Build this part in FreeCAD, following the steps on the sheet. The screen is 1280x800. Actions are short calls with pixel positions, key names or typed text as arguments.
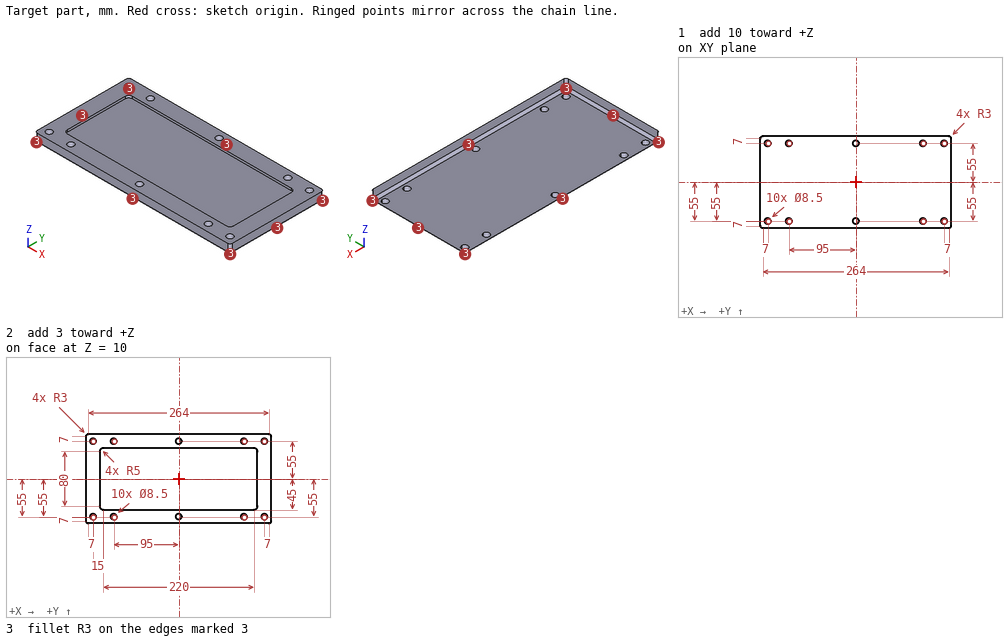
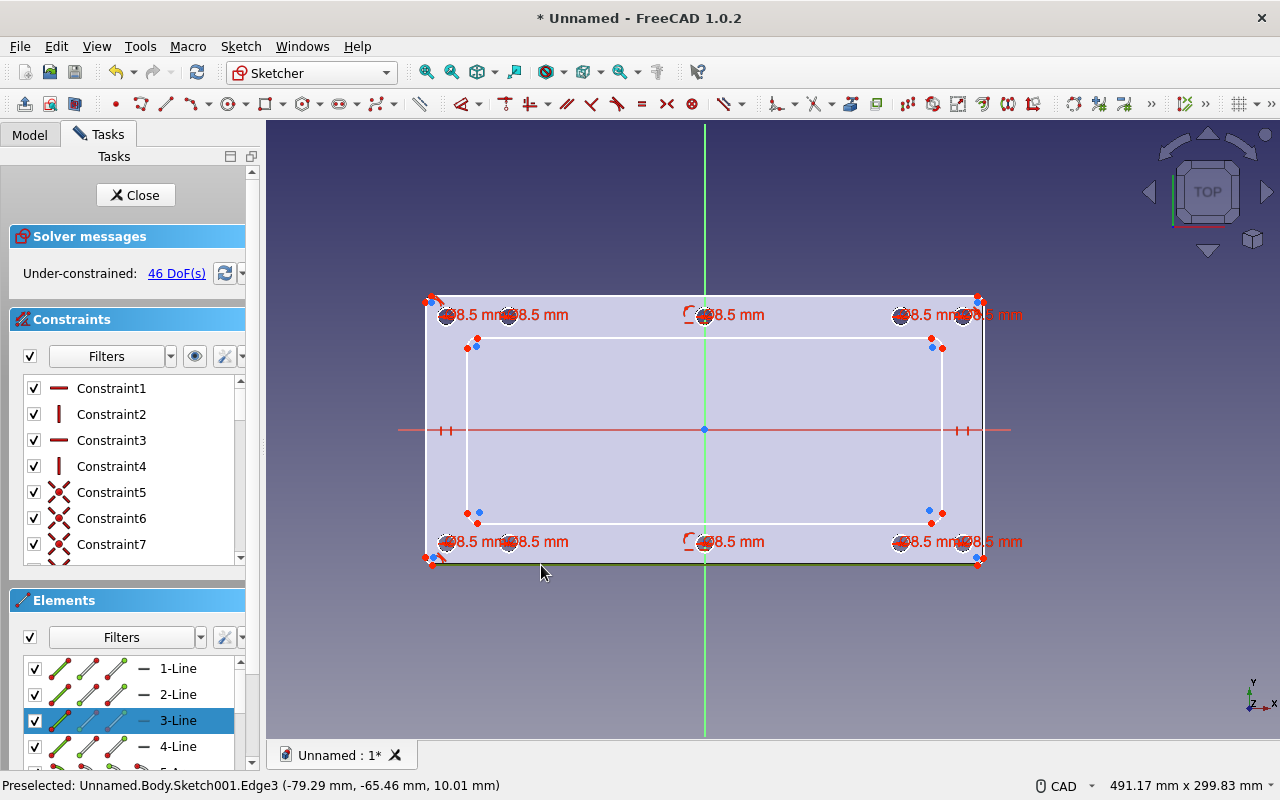
scroll(428, 563, up, 5)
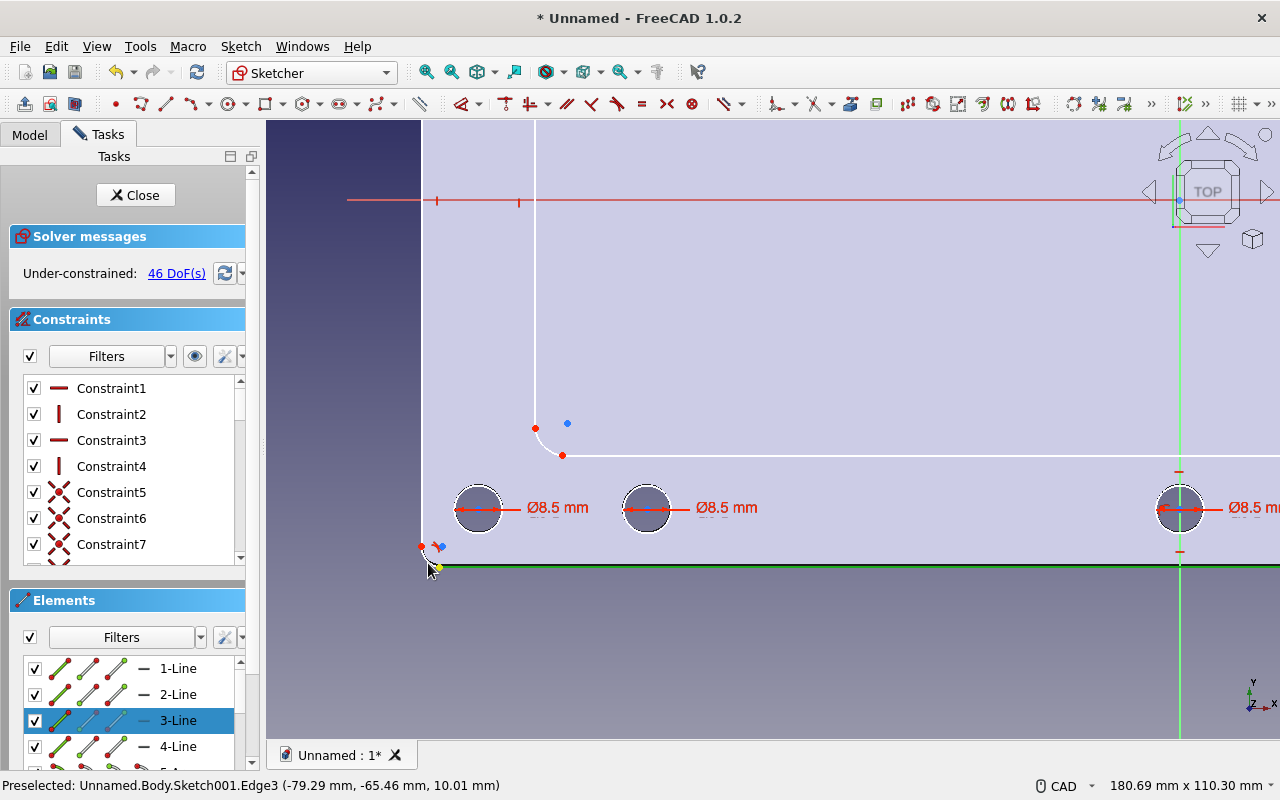
click(427, 560)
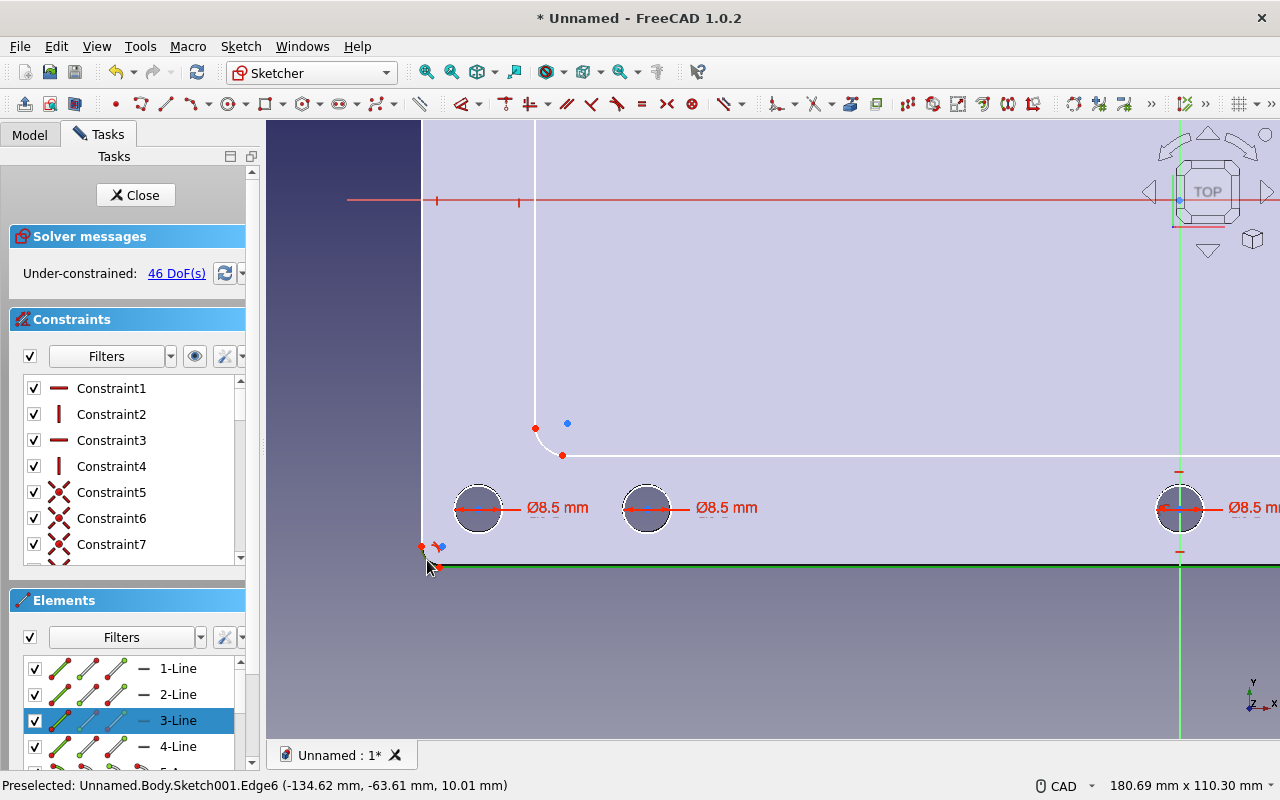
click(617, 104)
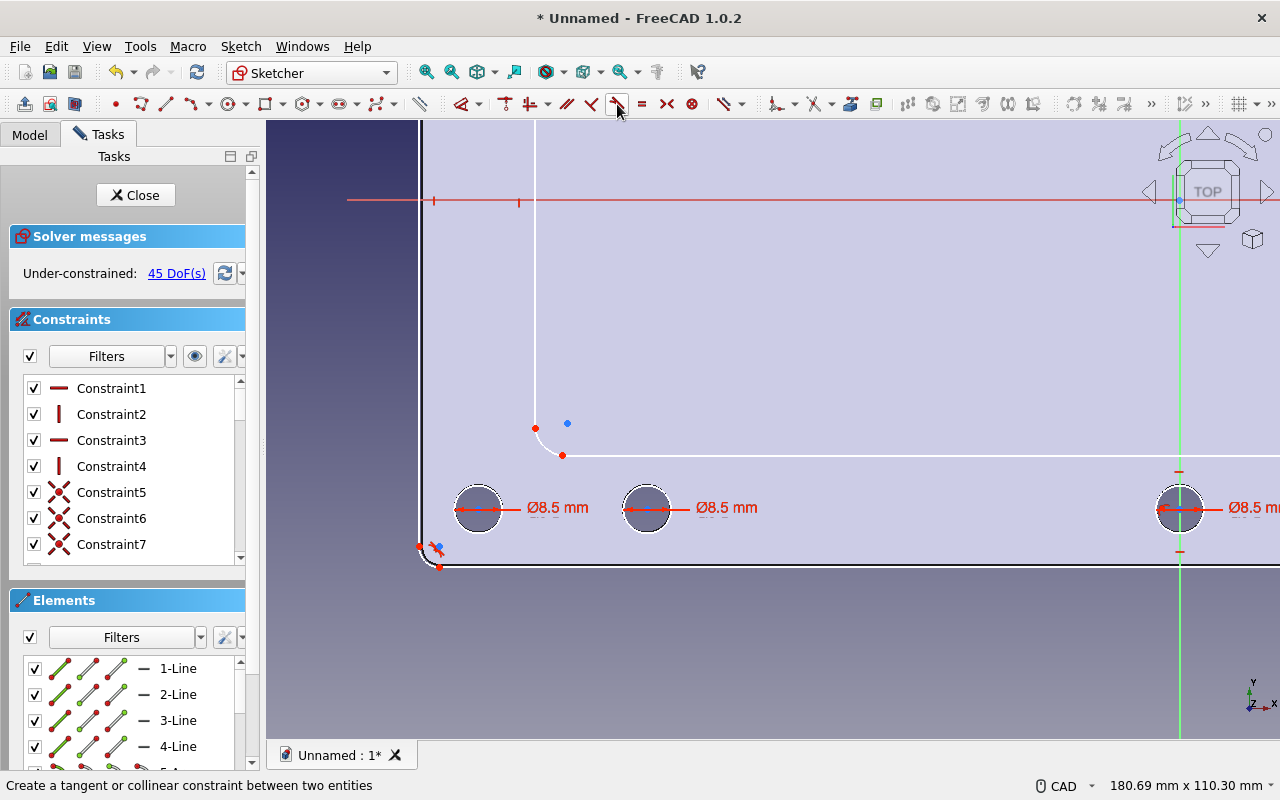
click(884, 567)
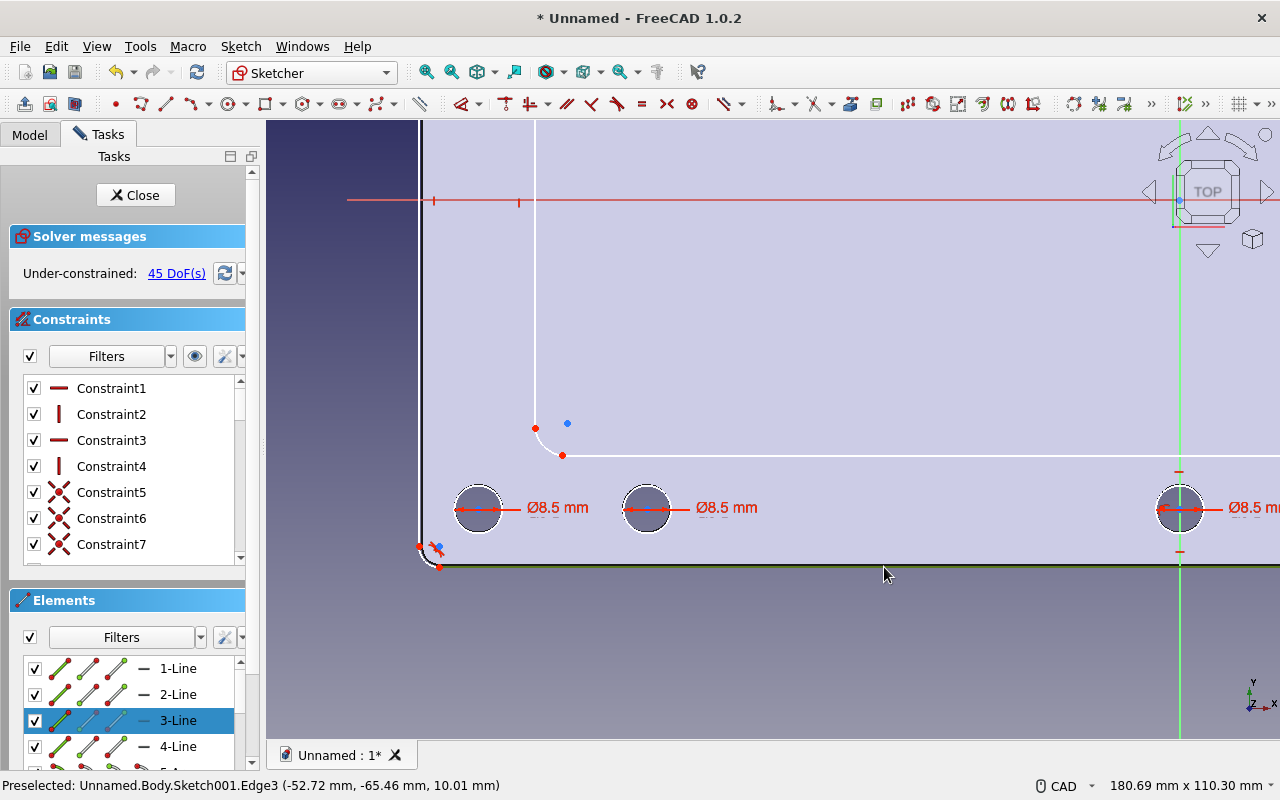
scroll(428, 563, down, 5)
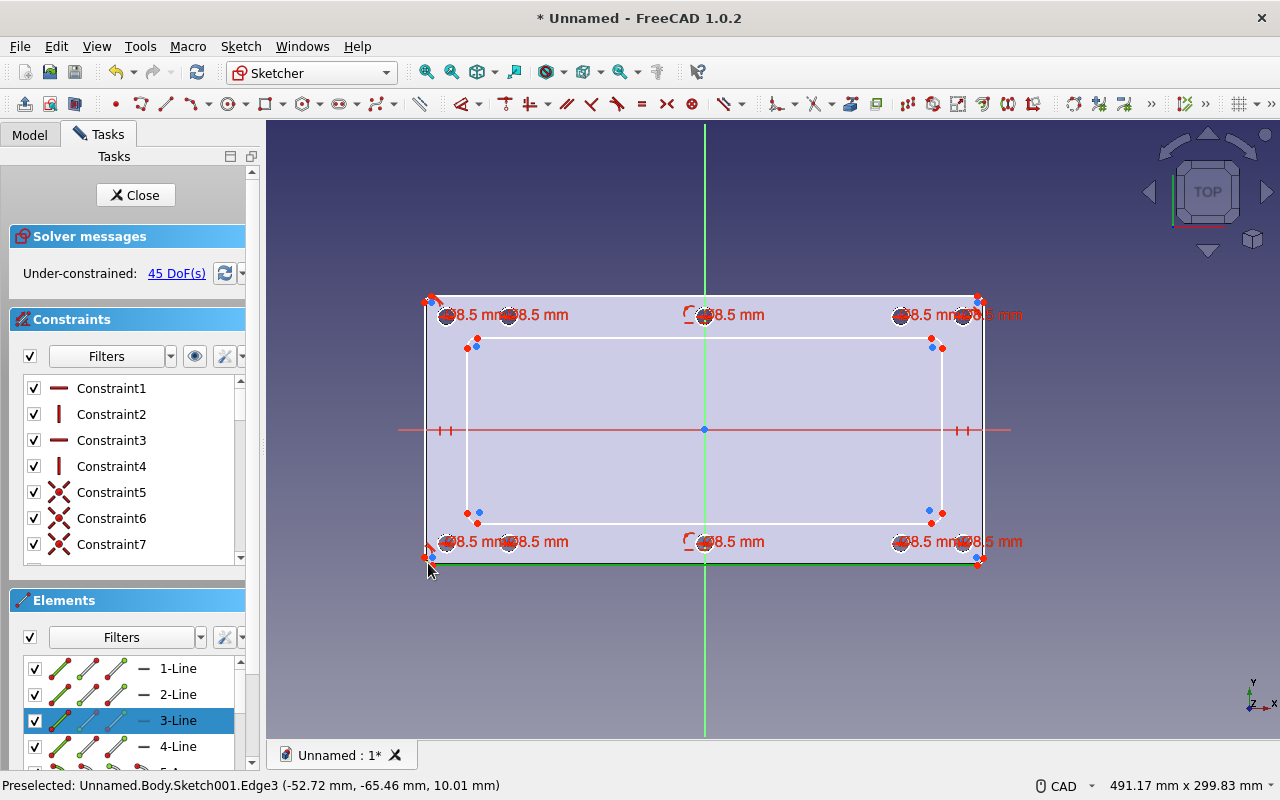
scroll(982, 563, up, 6)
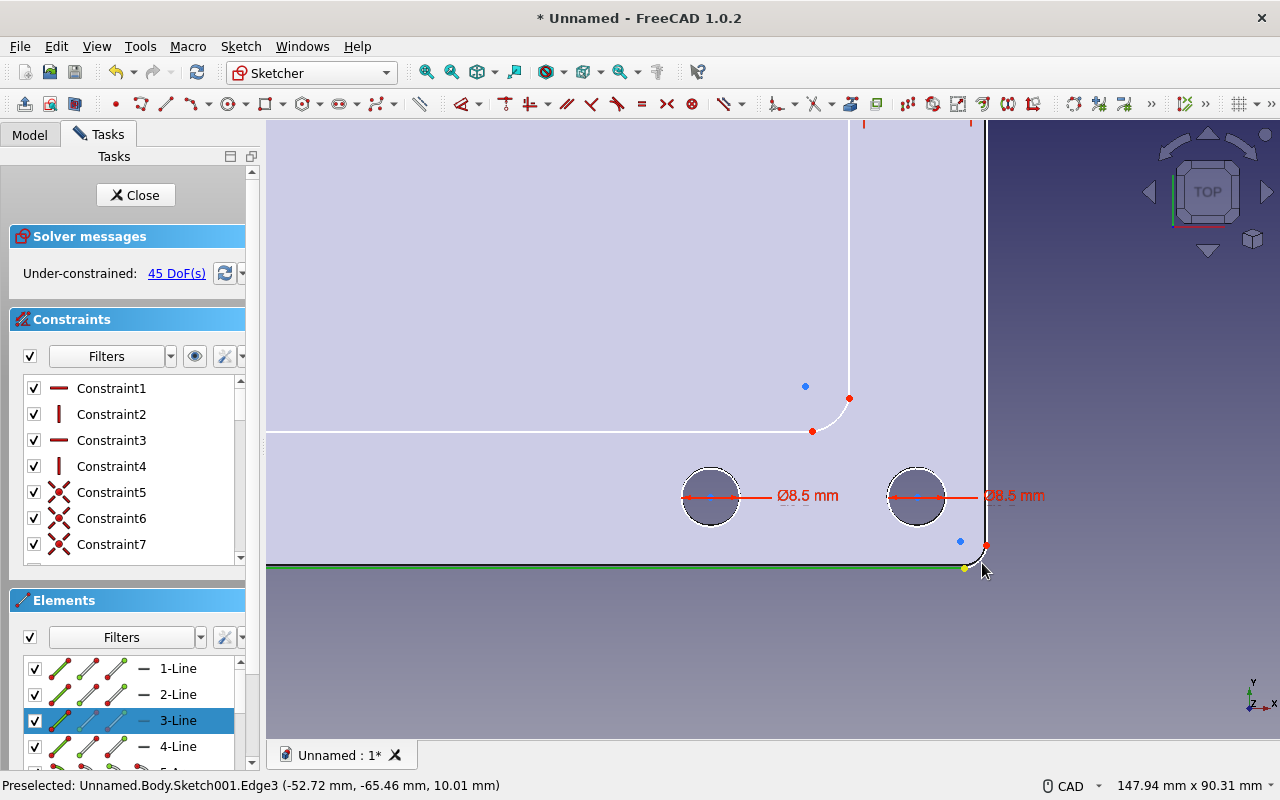
click(980, 561)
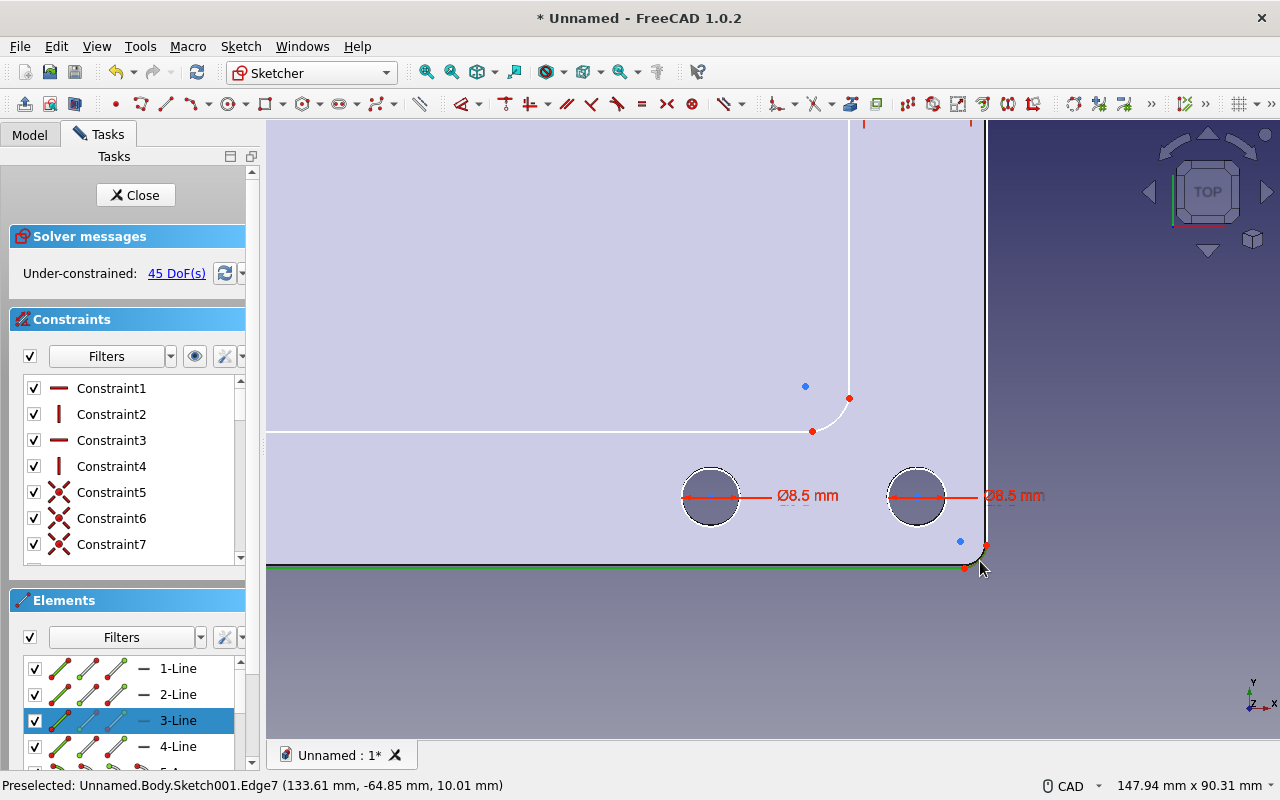
click(617, 104)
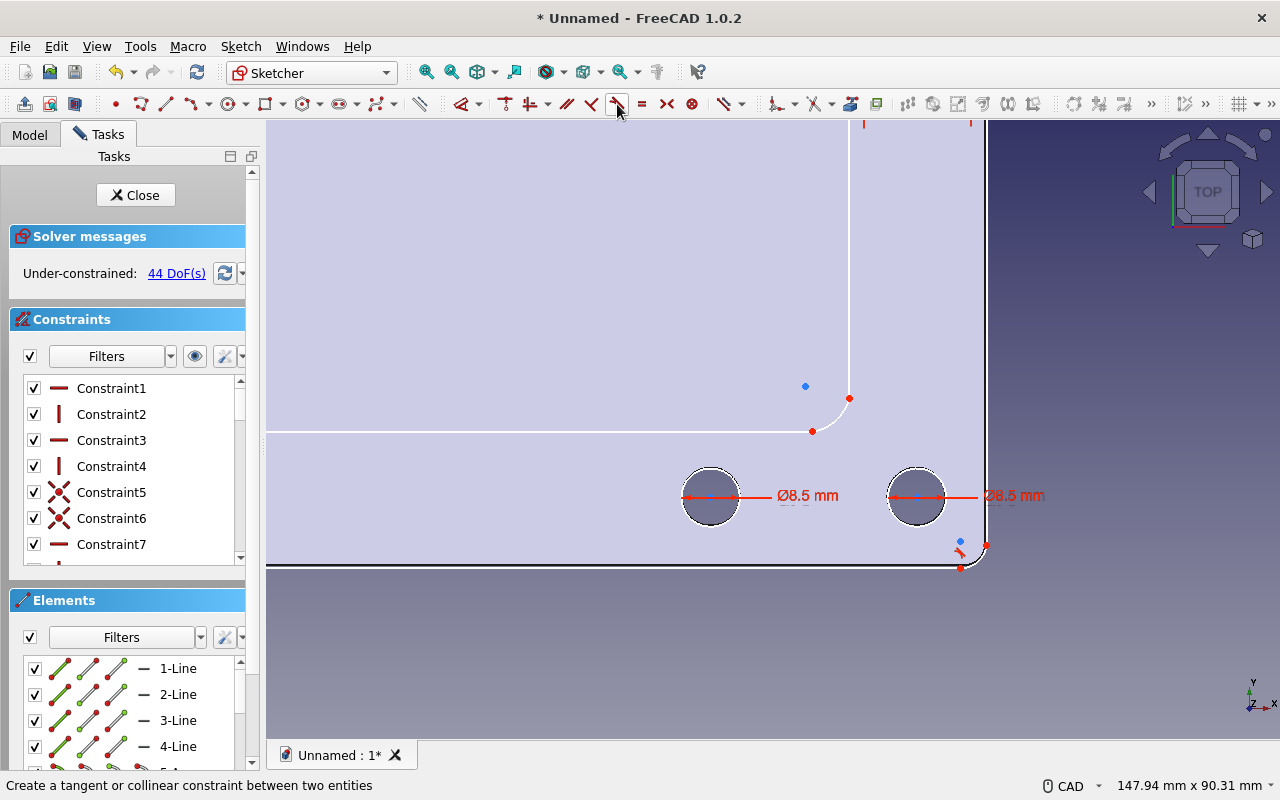
click(987, 291)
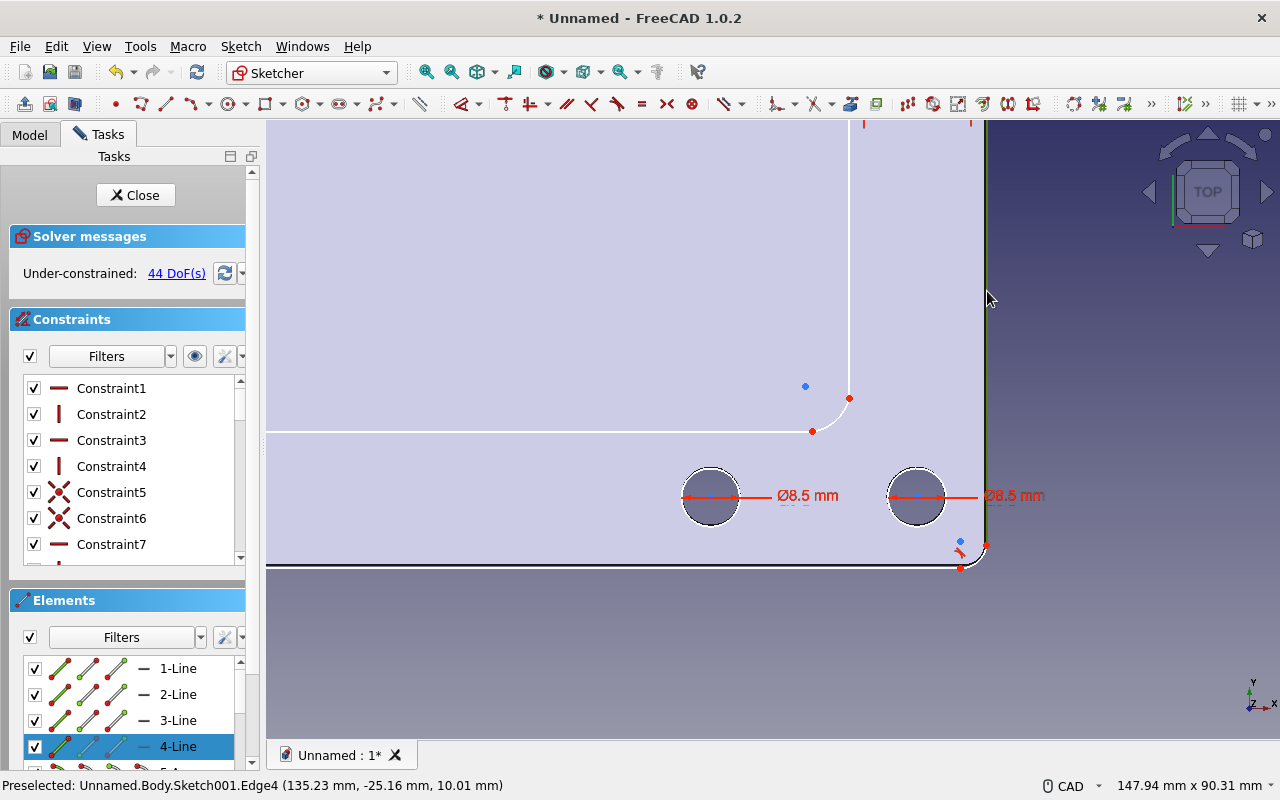
scroll(971, 566, up, 2)